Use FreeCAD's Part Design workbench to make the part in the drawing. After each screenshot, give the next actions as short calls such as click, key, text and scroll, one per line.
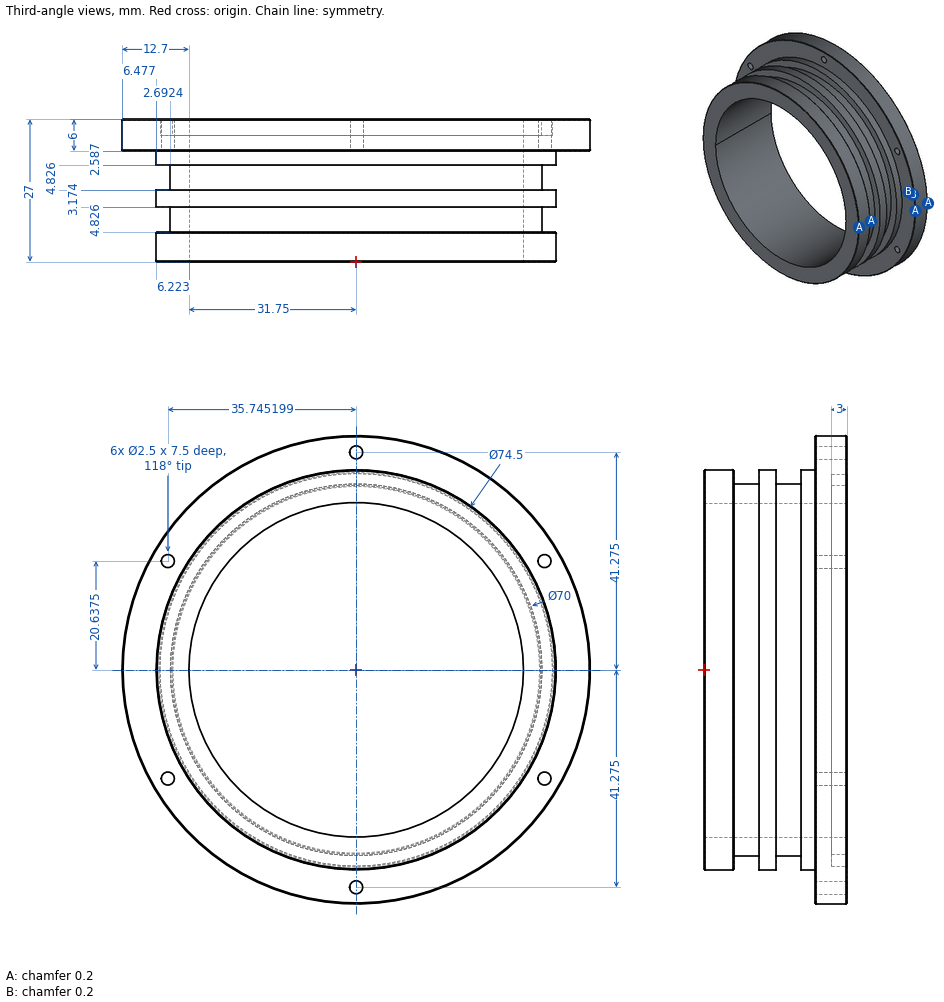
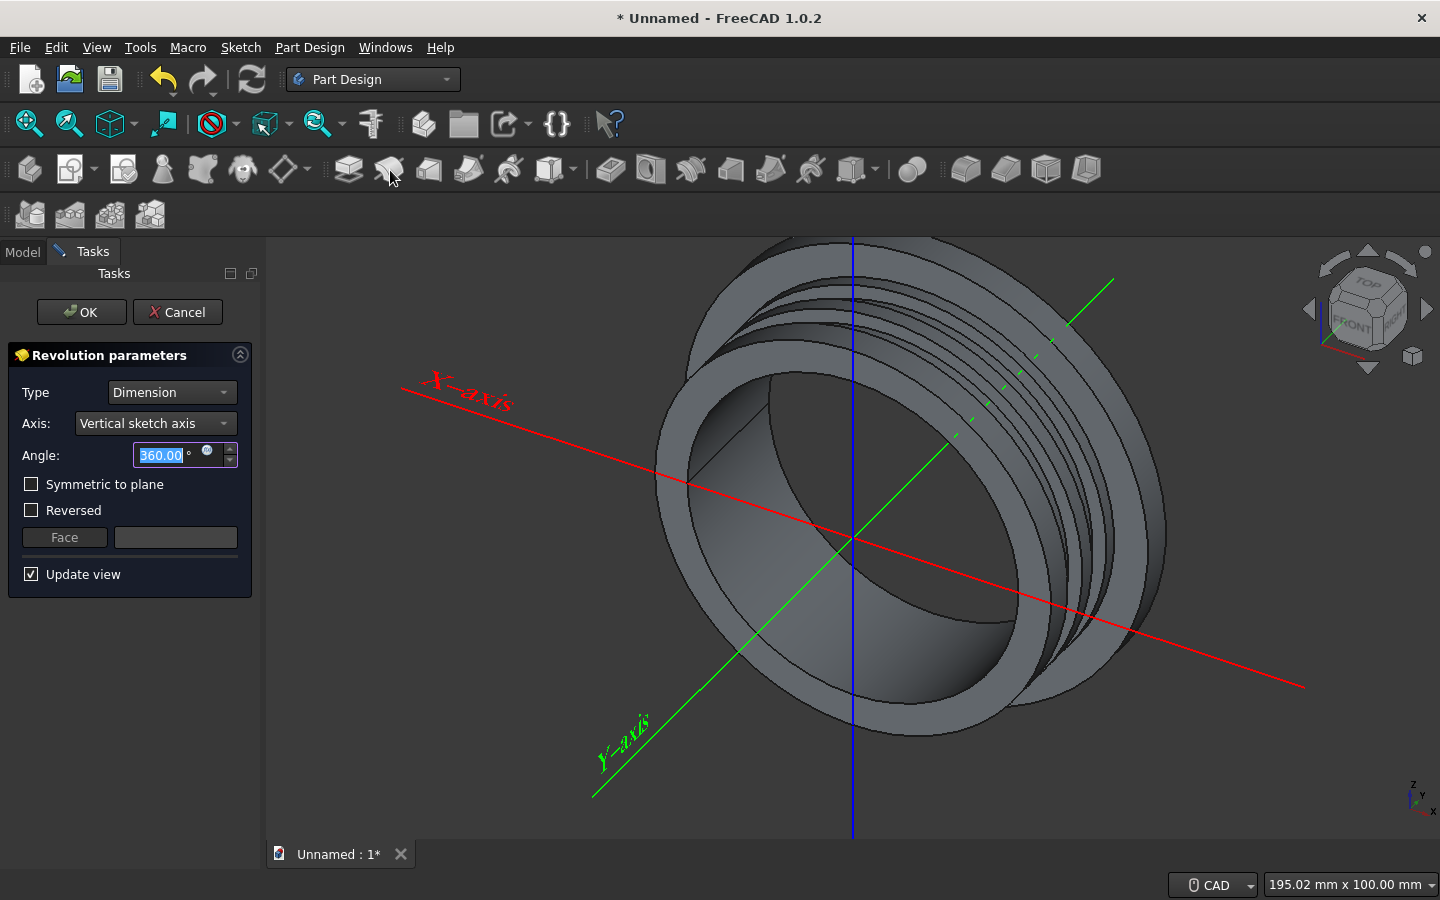
click(82, 312)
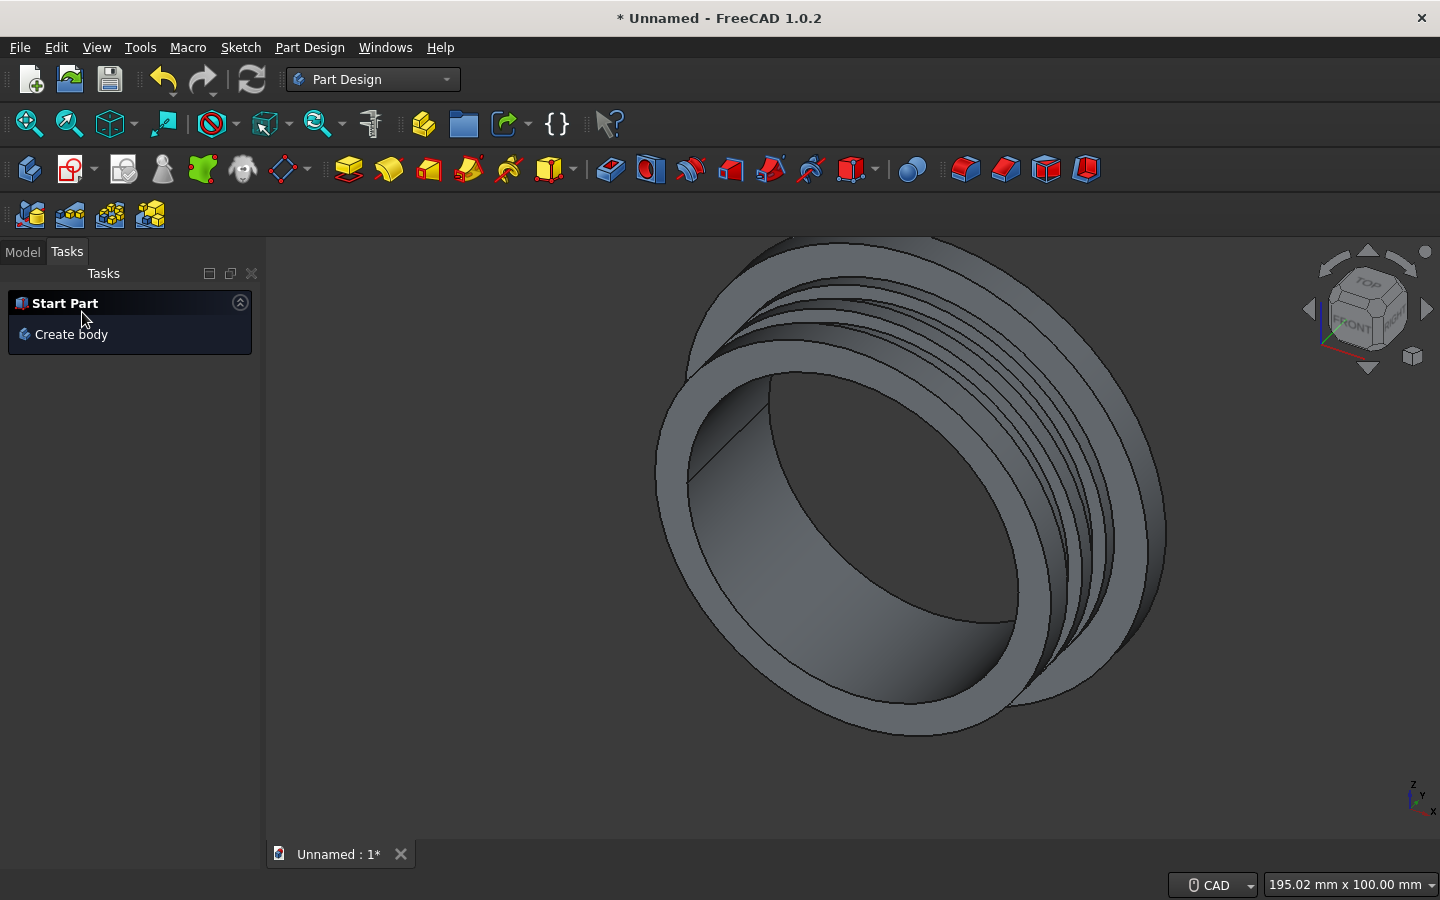
key(v)
key(f)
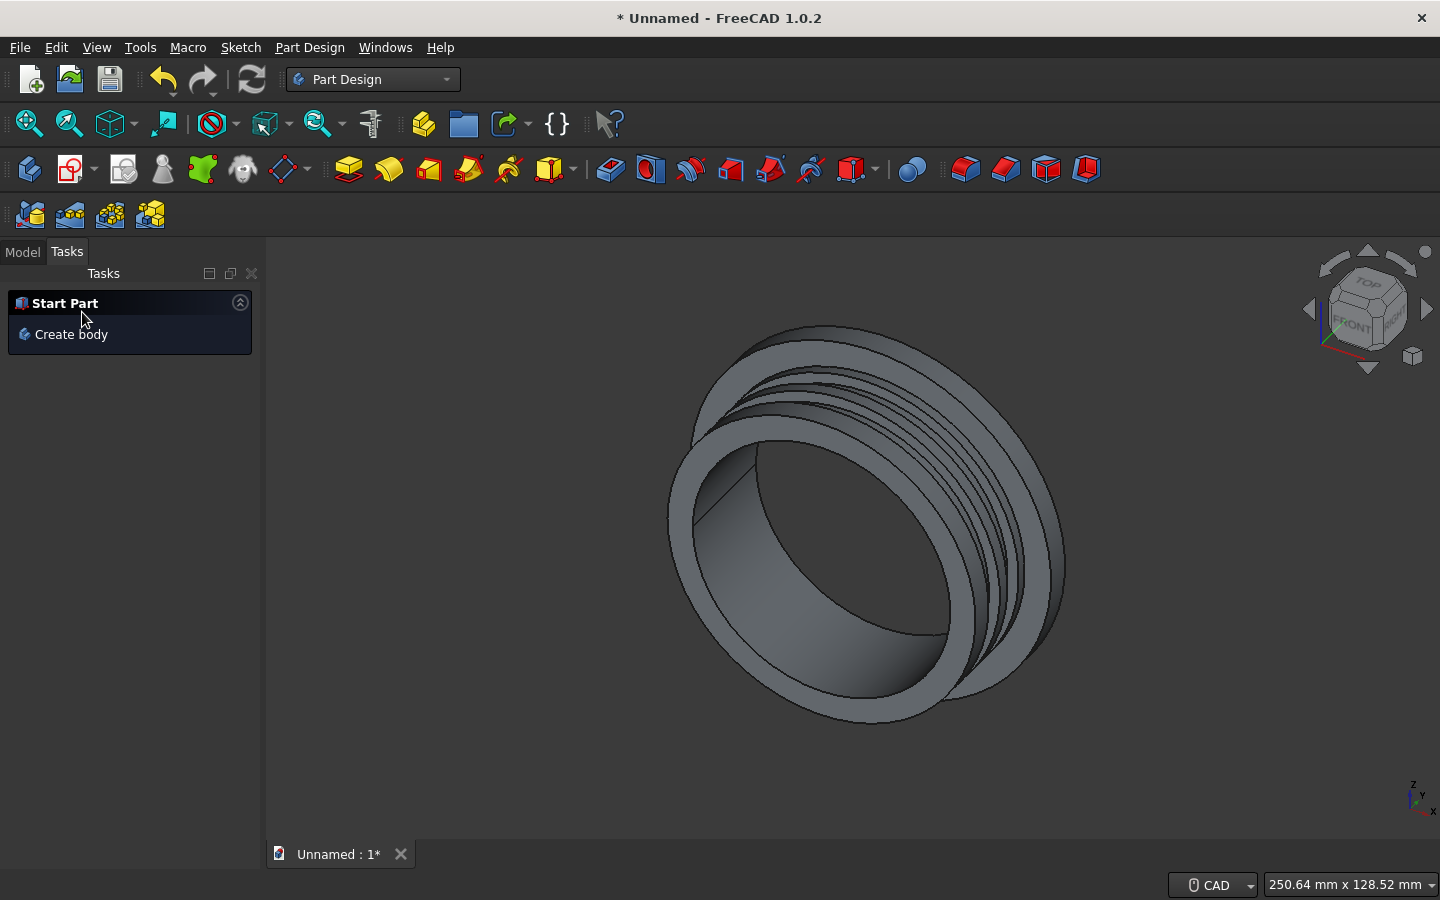
click(976, 619)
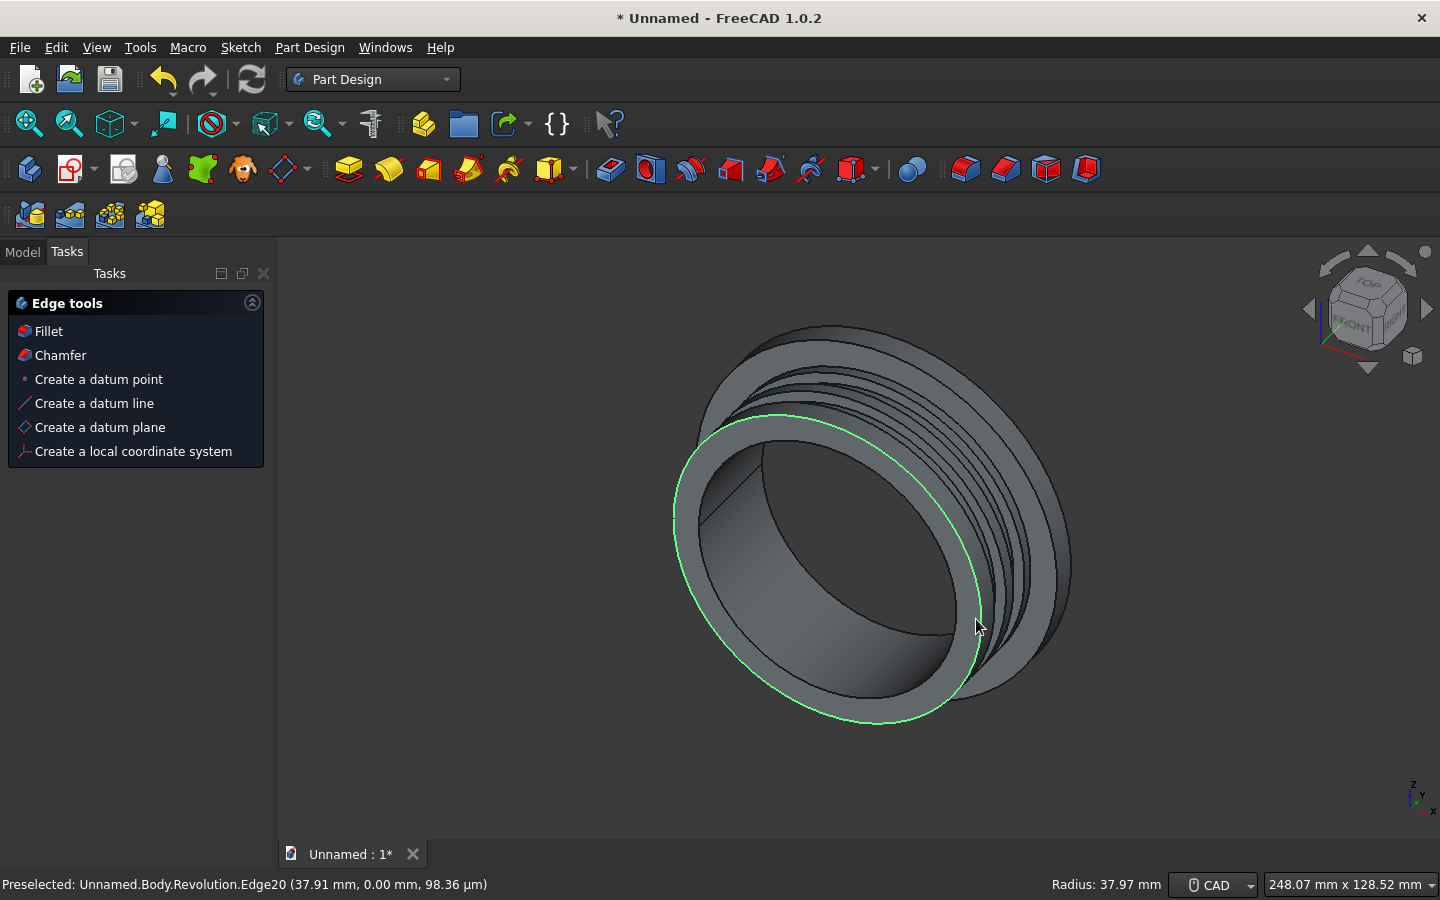
click(1057, 579, ctrl)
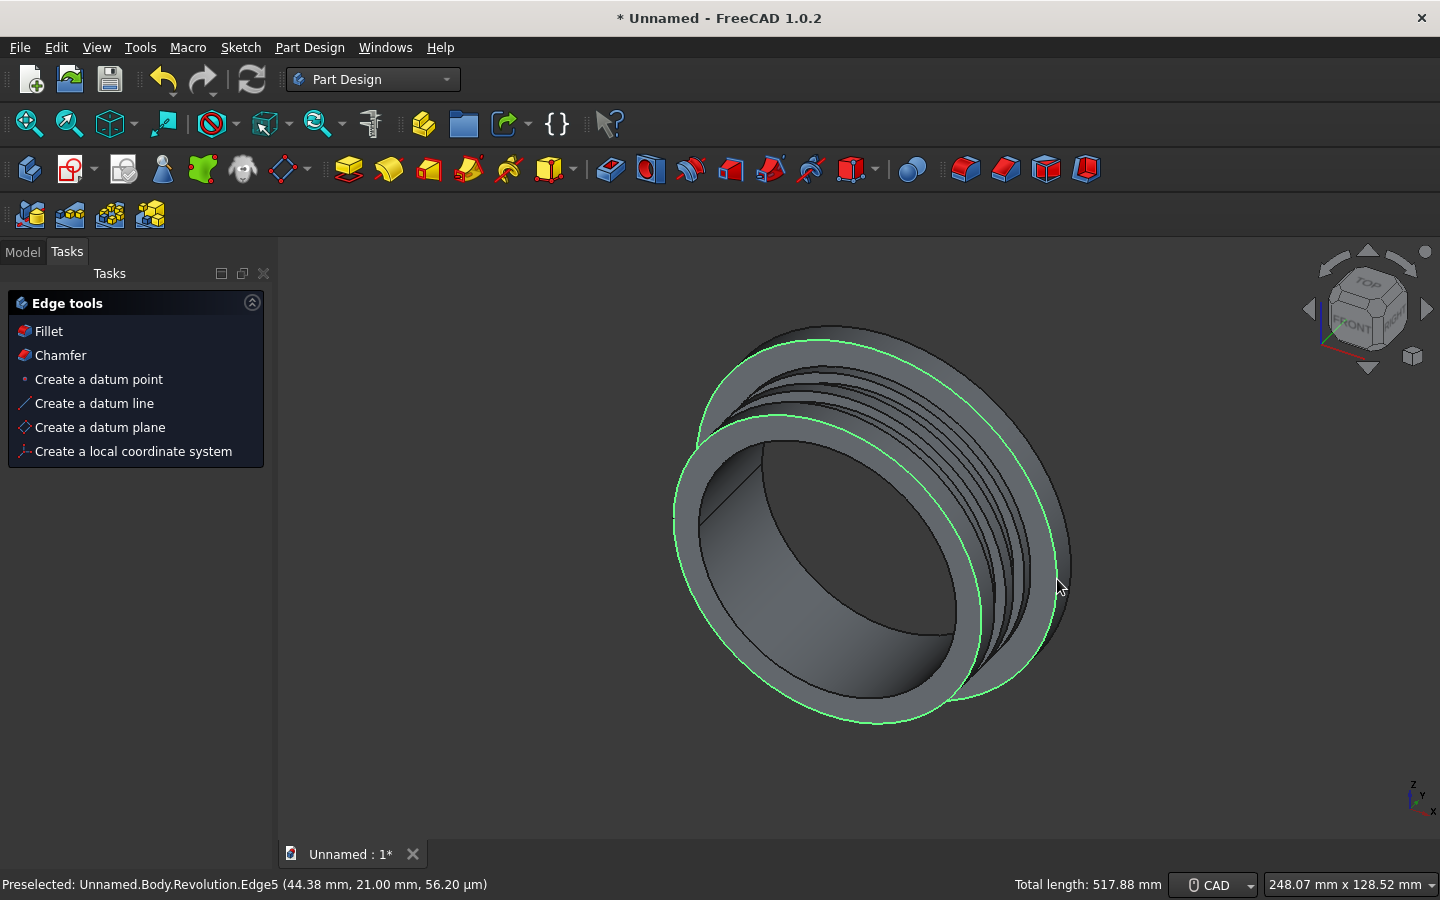
key(0)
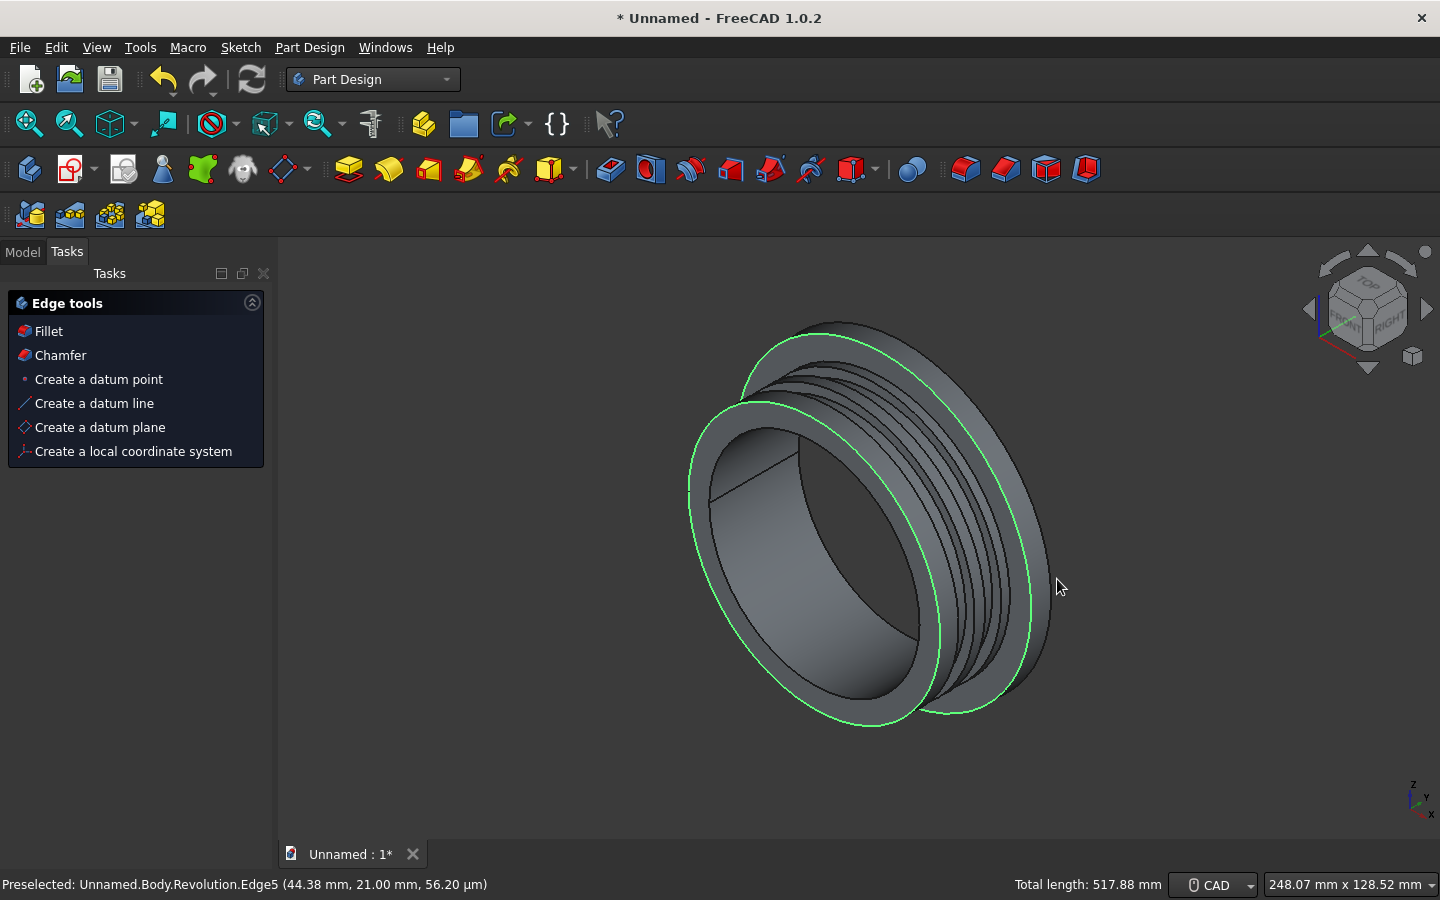
key(2)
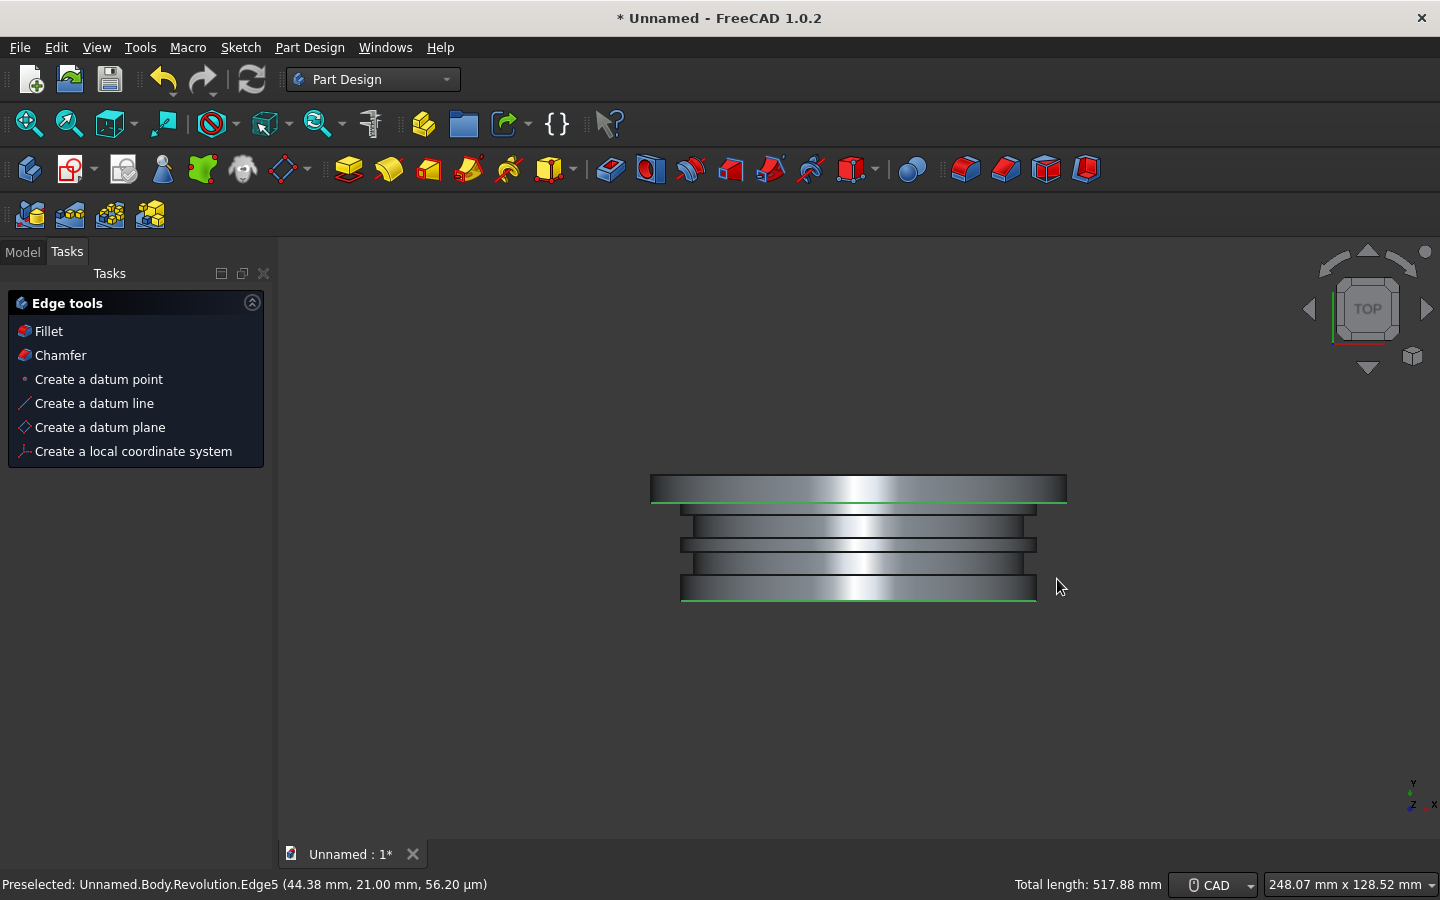
key(v)
key(f)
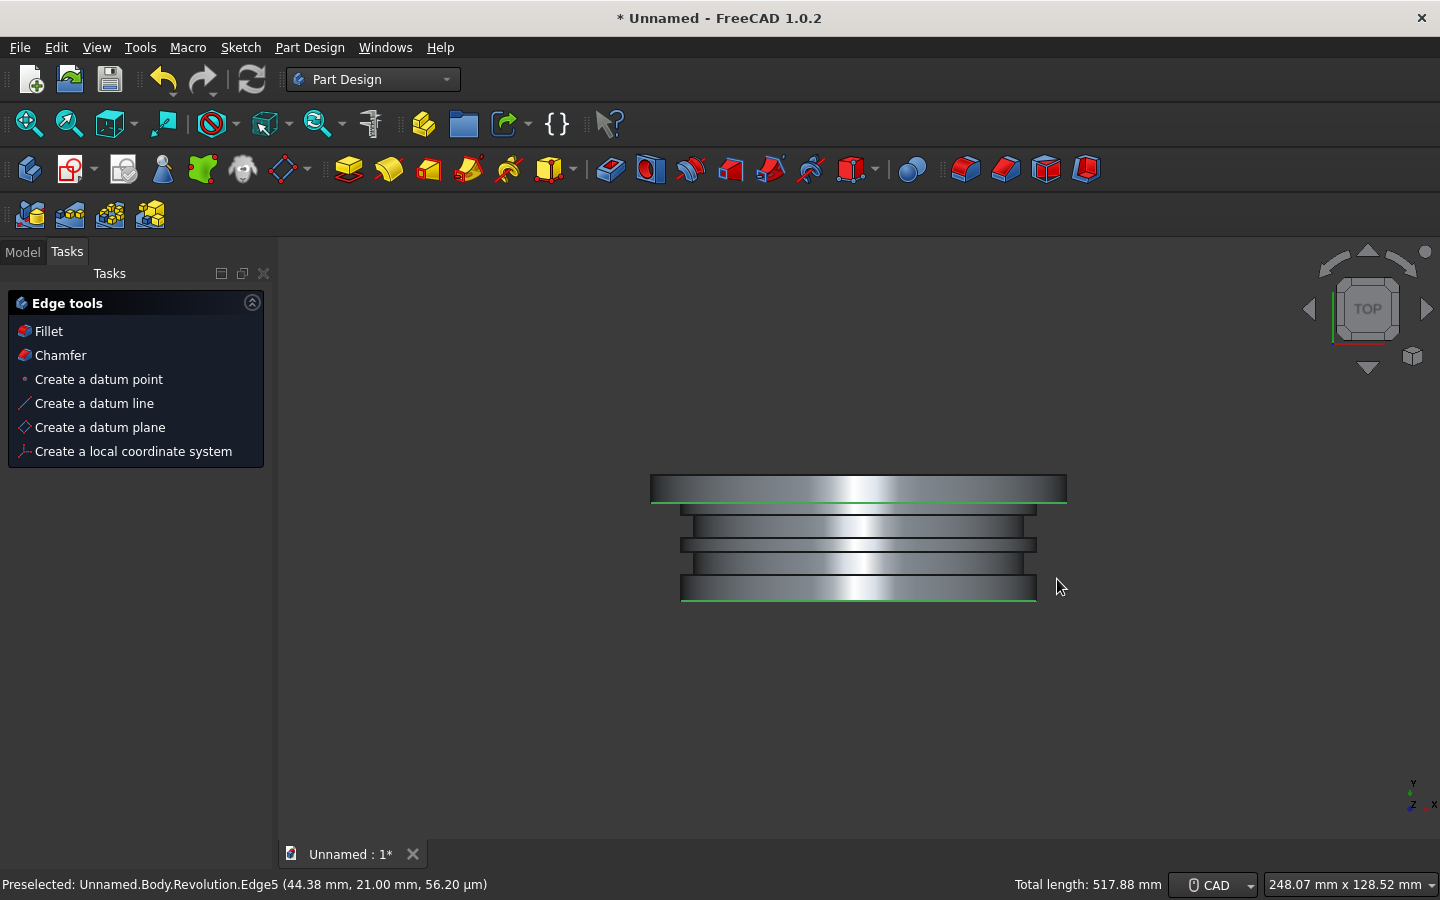
click(1003, 574, ctrl)